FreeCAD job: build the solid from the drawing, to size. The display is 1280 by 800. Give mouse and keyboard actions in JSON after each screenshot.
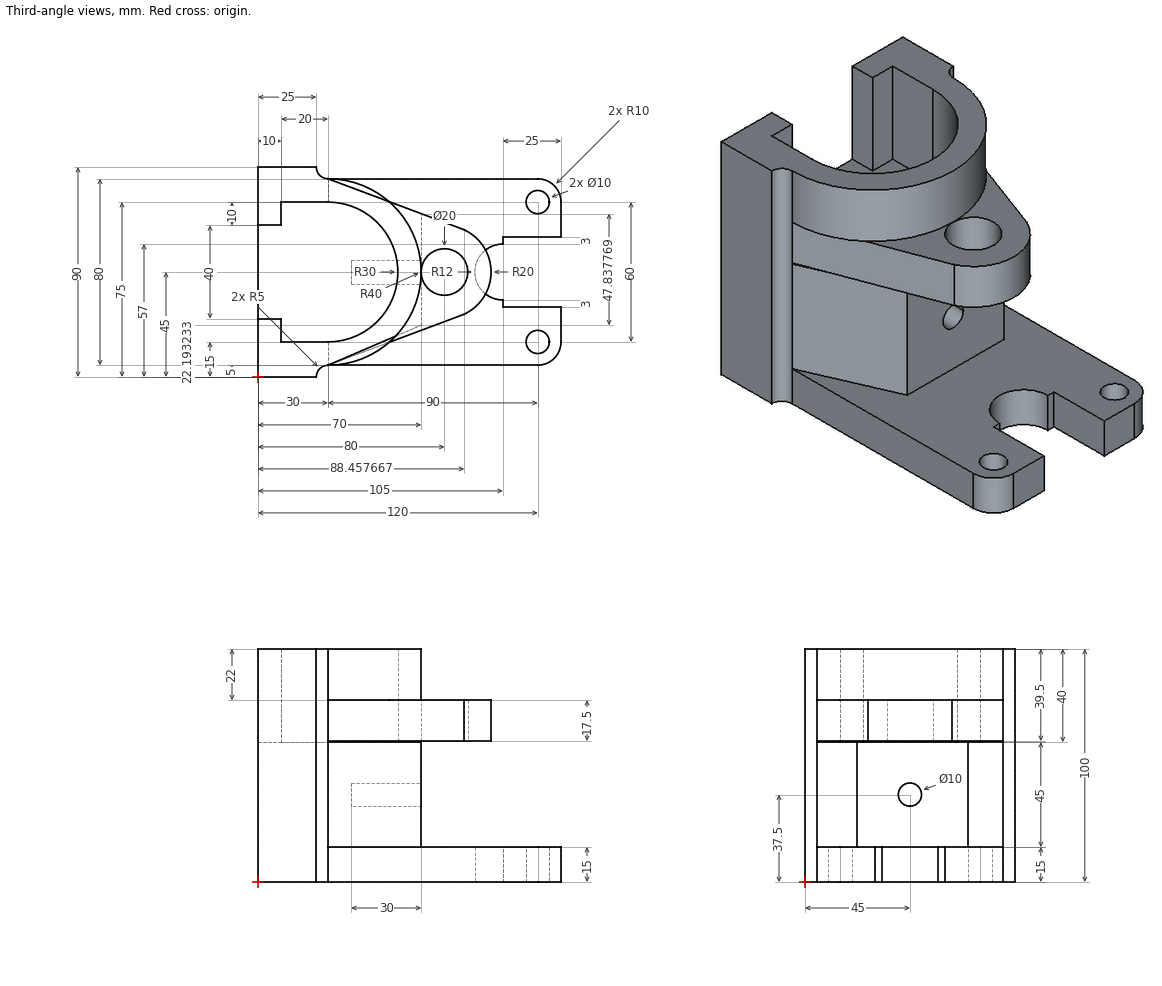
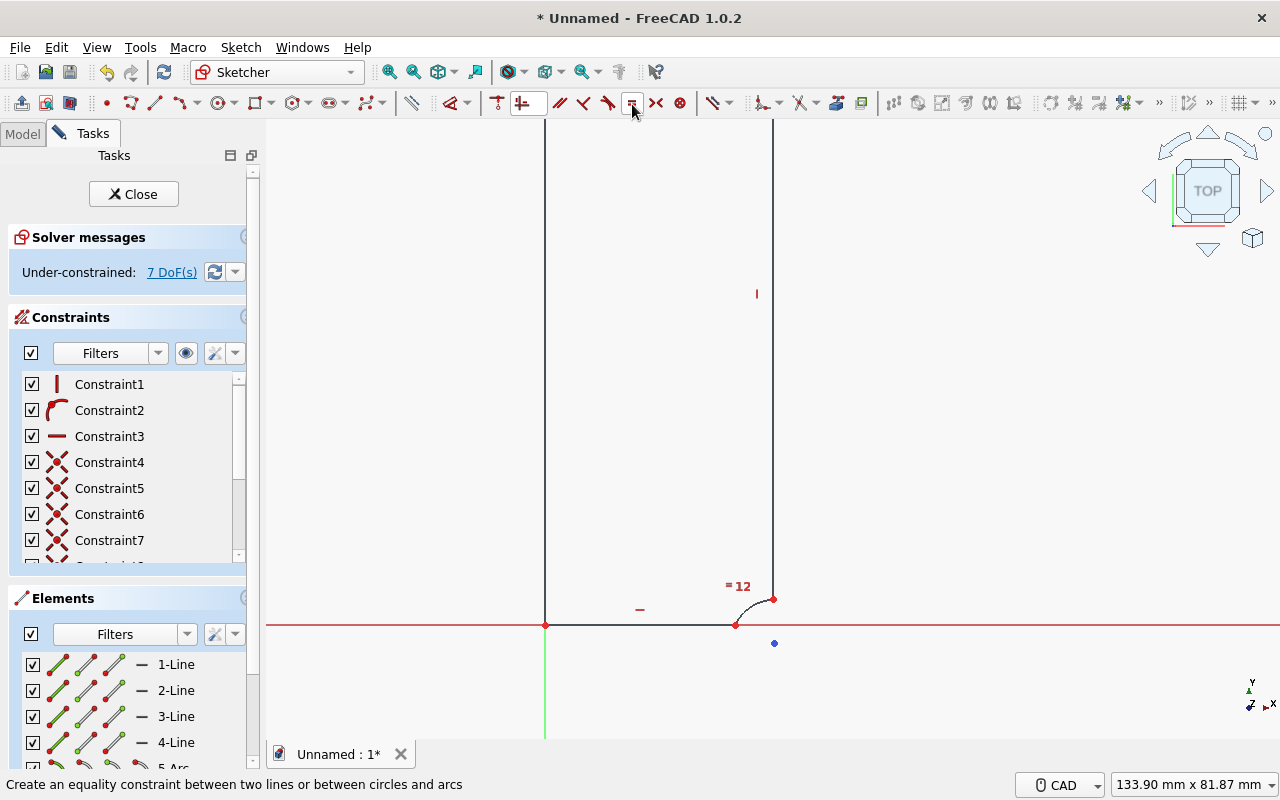
{"action": "left_click", "coordinate": [775, 644]}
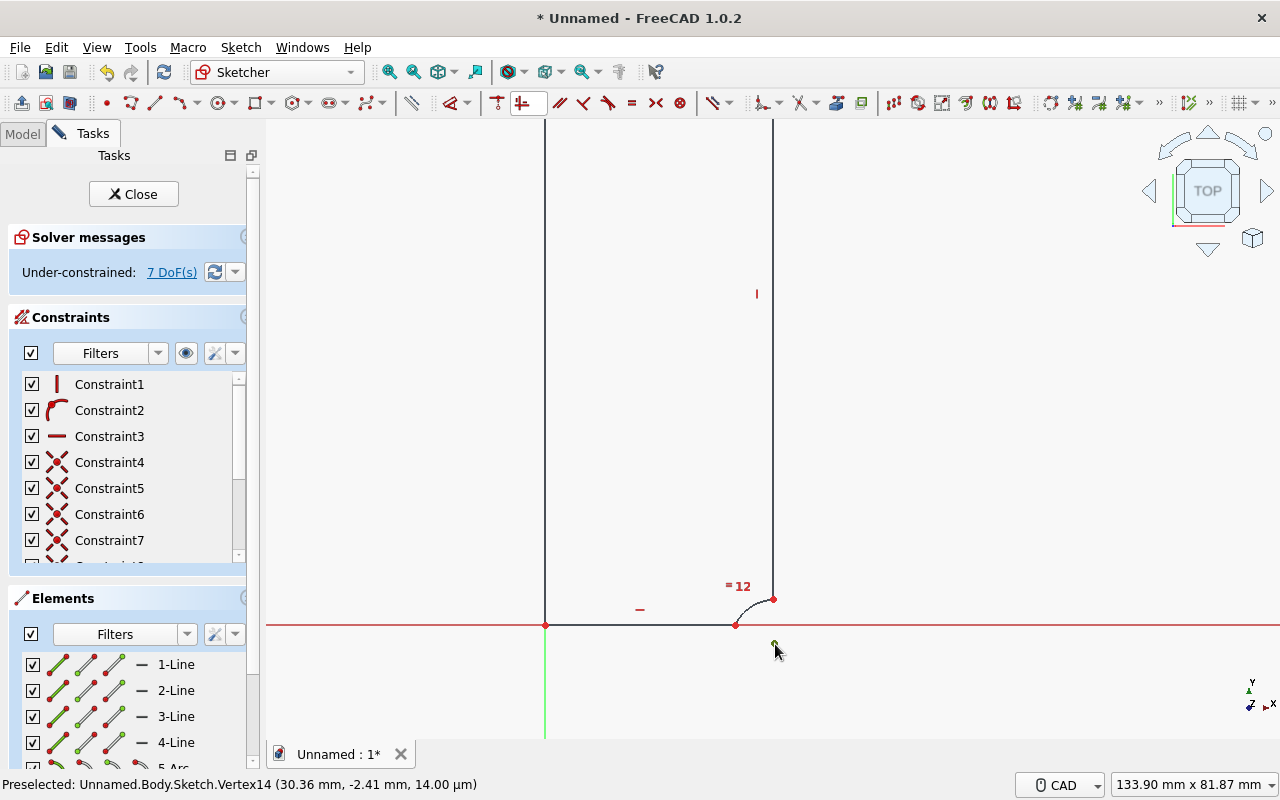
{"action": "left_click", "coordinate": [353, 625]}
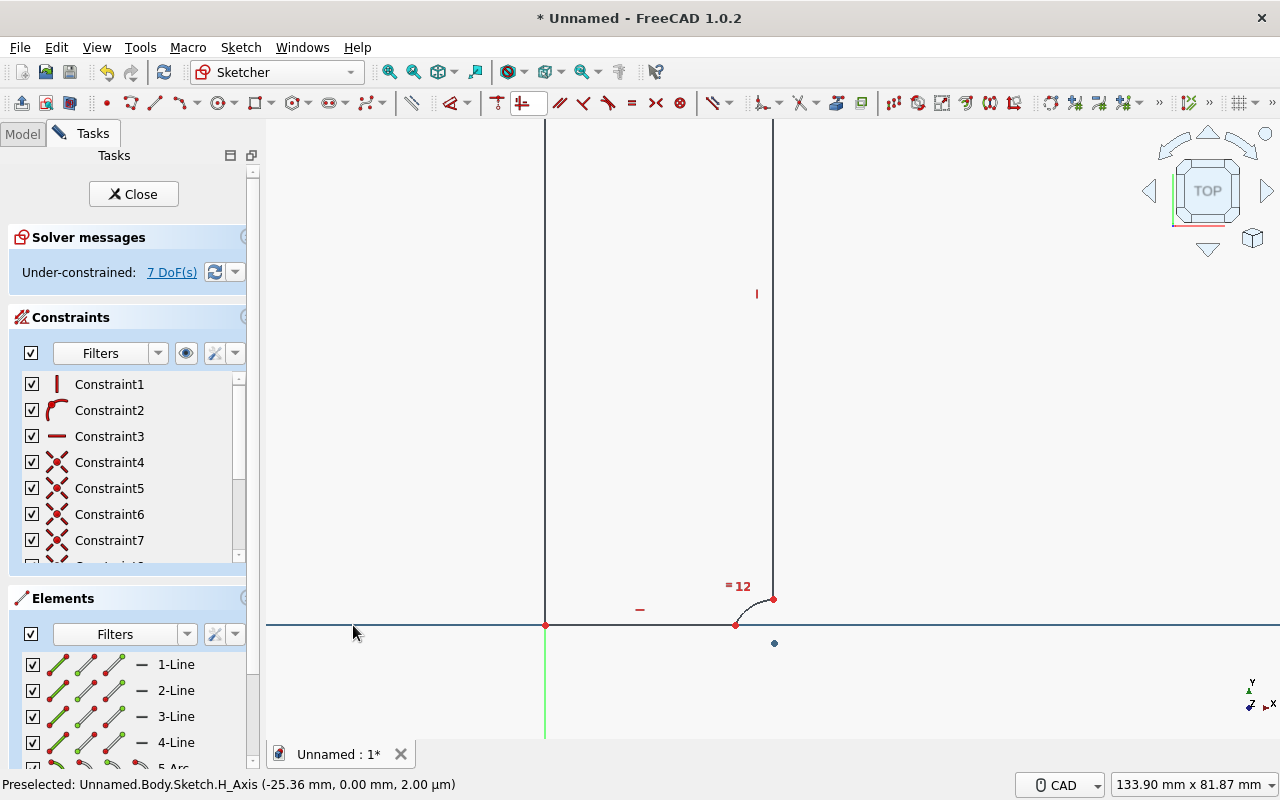
{"action": "left_click", "coordinate": [498, 104]}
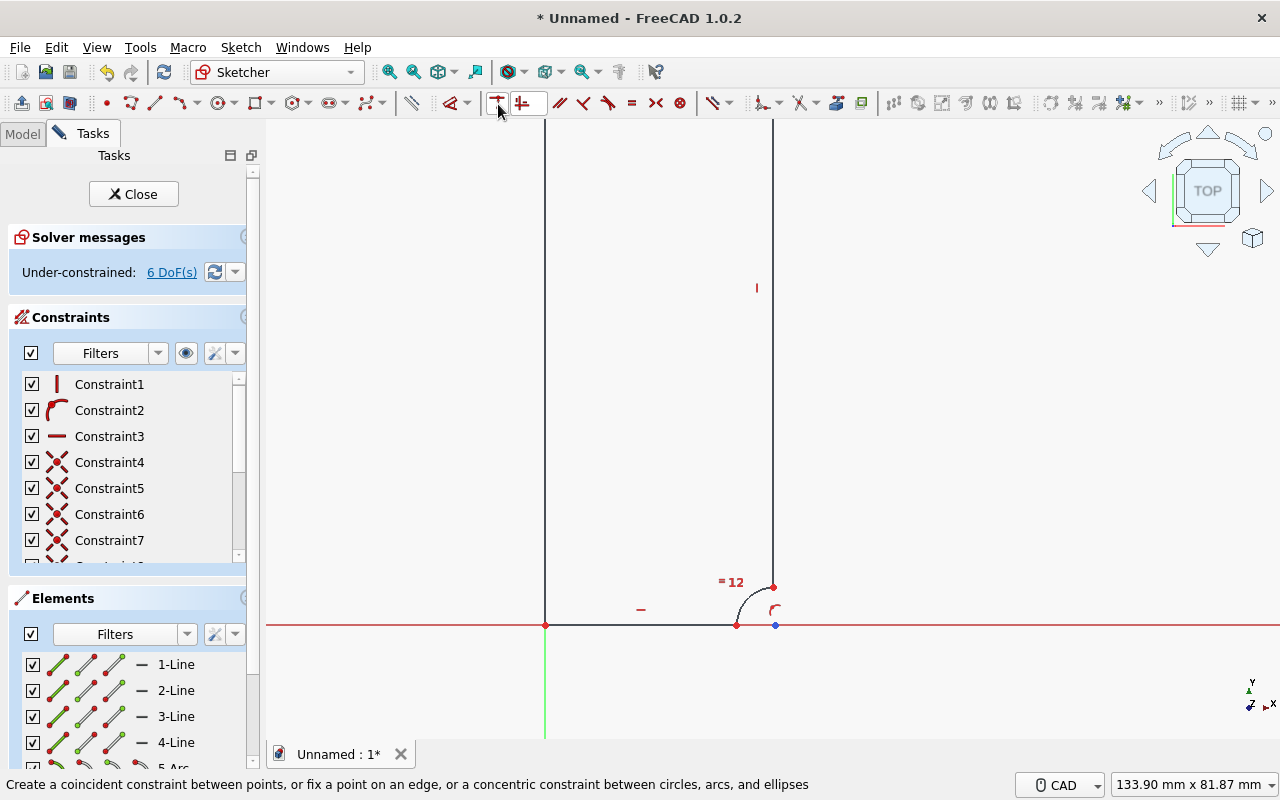
{"action": "key", "text": "d"}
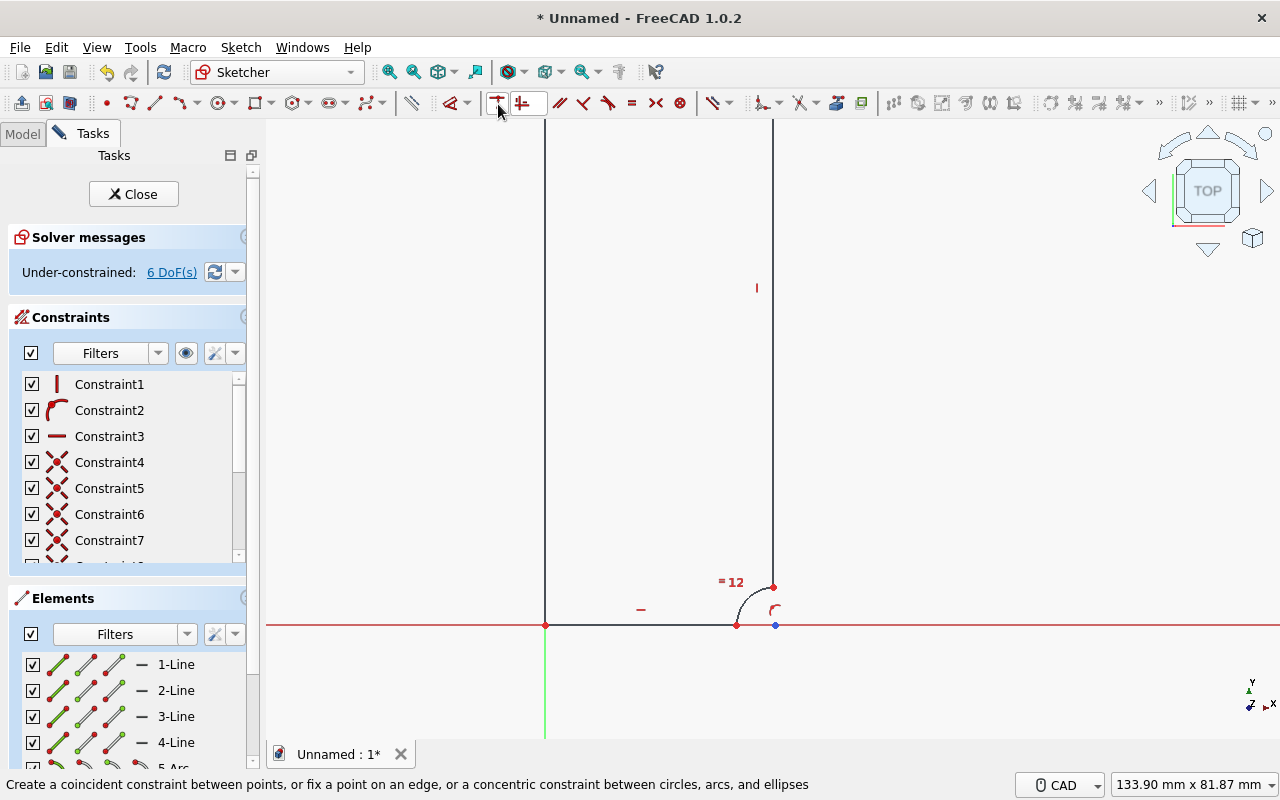
{"action": "scroll", "coordinate": [760, 605], "scroll_direction": "down", "scroll_amount": 3}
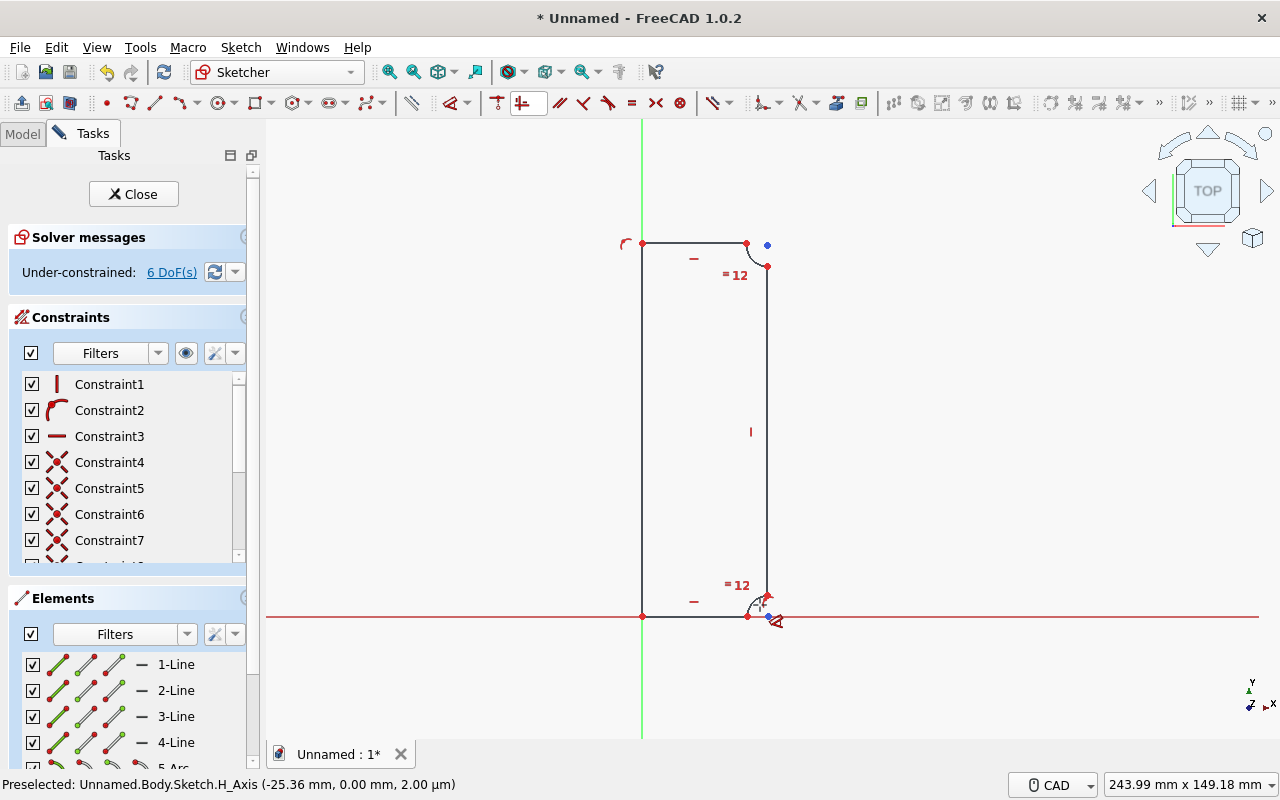
{"action": "scroll", "coordinate": [748, 254], "scroll_direction": "up", "scroll_amount": 4}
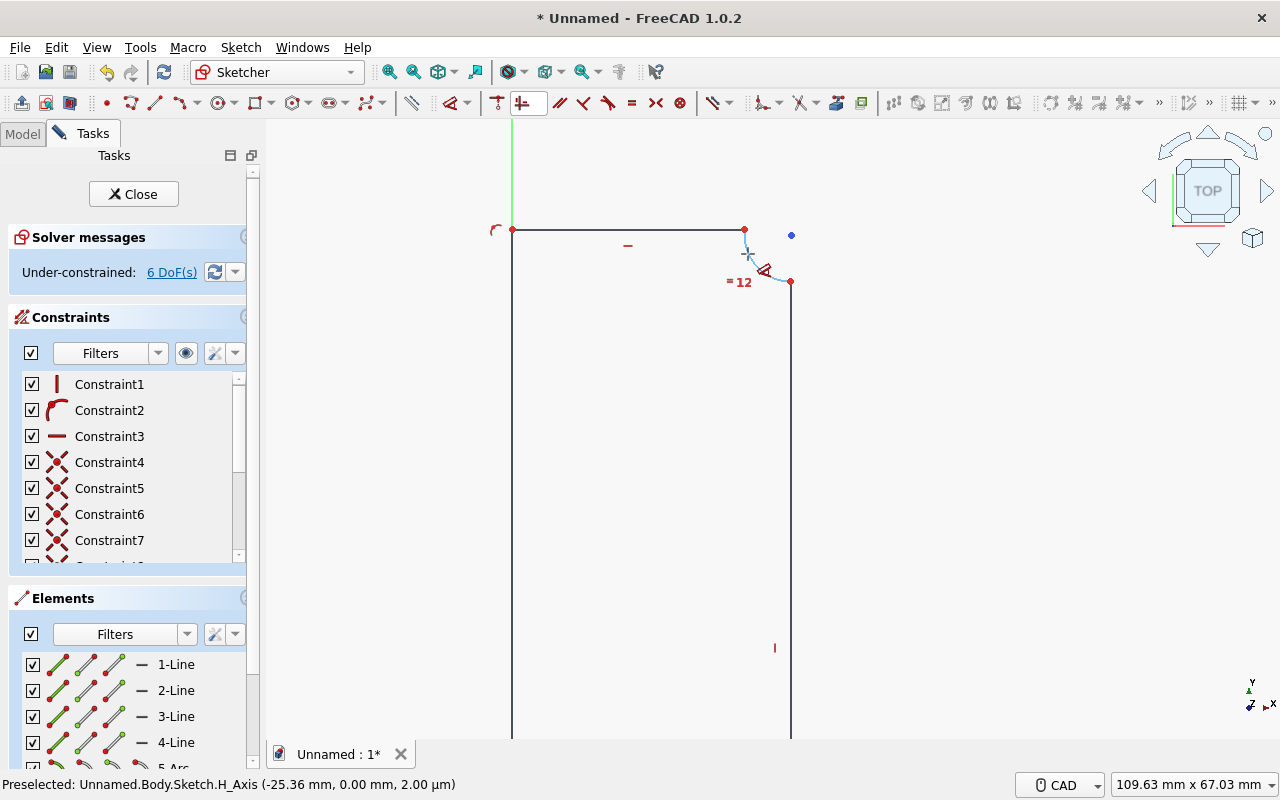
{"action": "left_click", "coordinate": [748, 253]}
{"action": "left_click", "coordinate": [718, 265]}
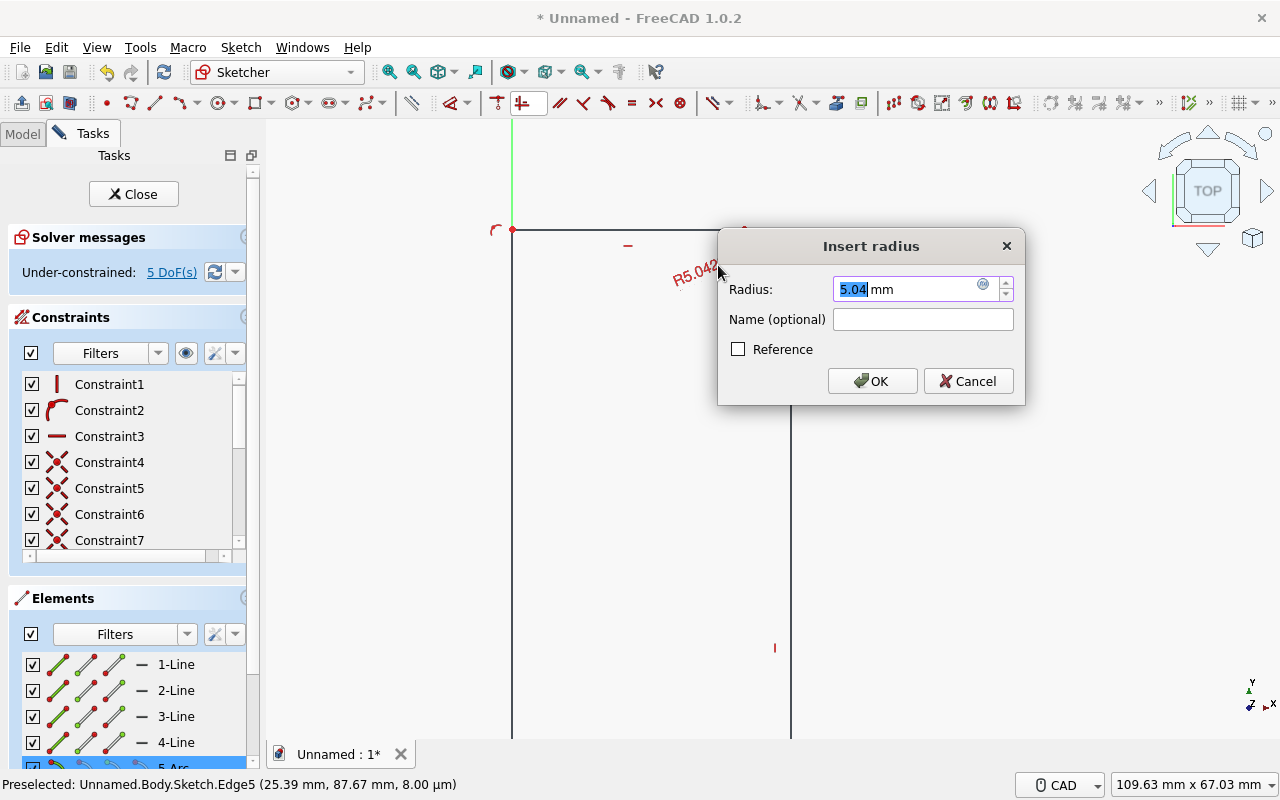
{"action": "type", "text": "5"}
{"action": "key", "text": "Return"}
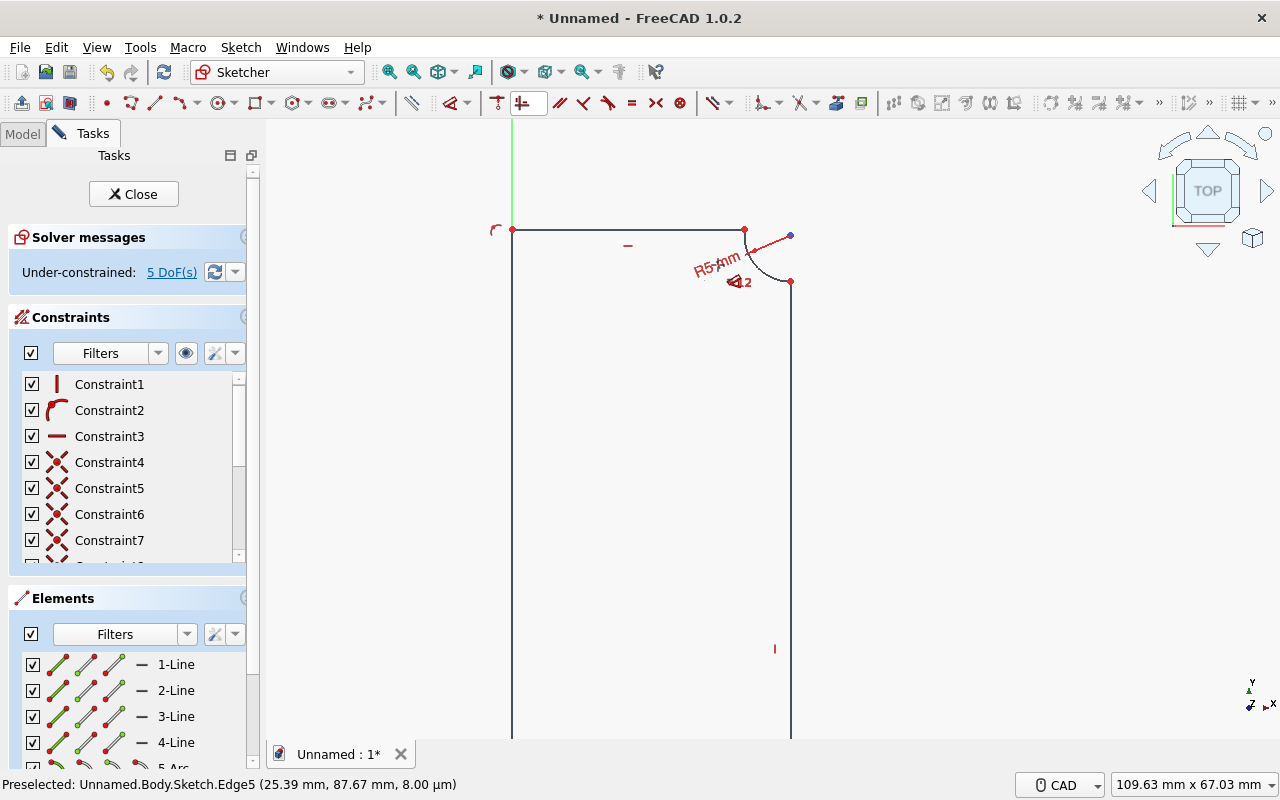
{"action": "left_click", "coordinate": [791, 502]}
{"action": "left_click", "coordinate": [825, 496]}